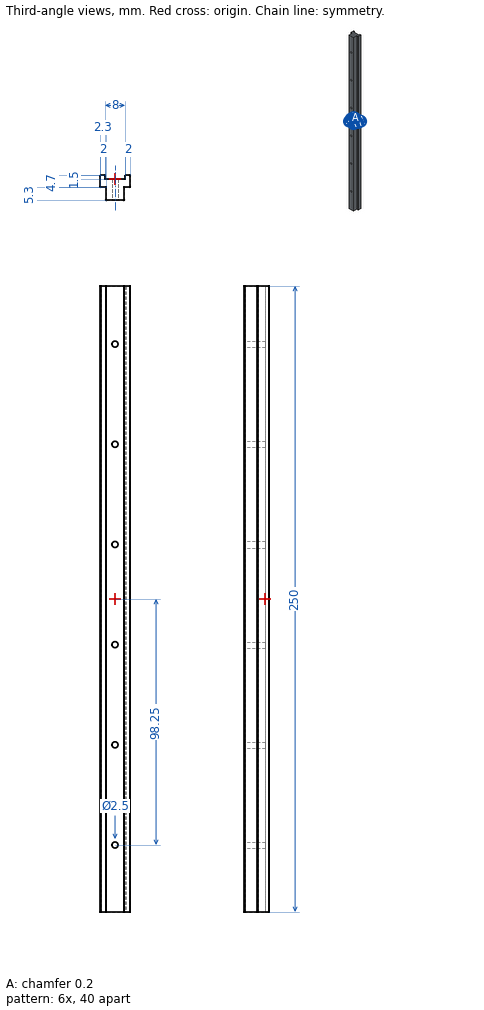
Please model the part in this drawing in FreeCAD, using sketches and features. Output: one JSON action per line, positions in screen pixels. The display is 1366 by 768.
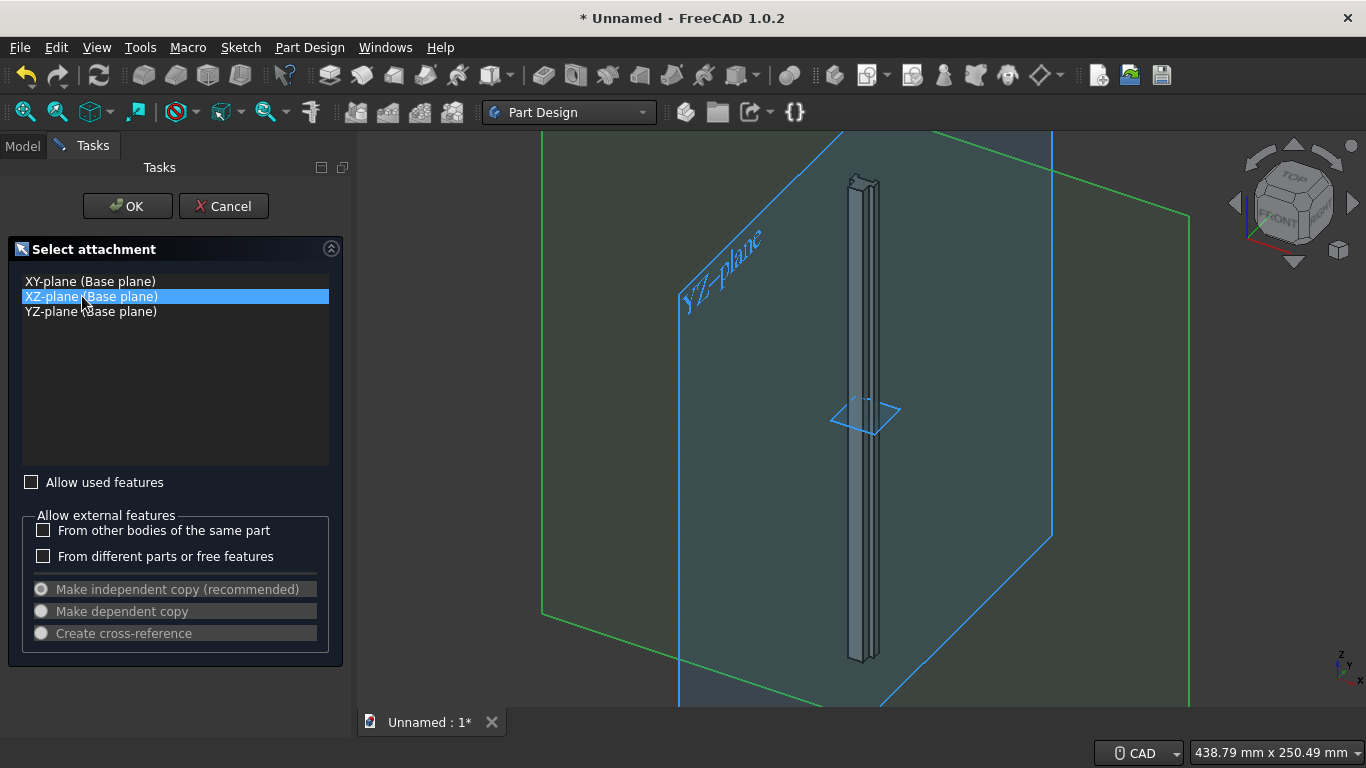
{"action": "left_click", "coordinate": [128, 206]}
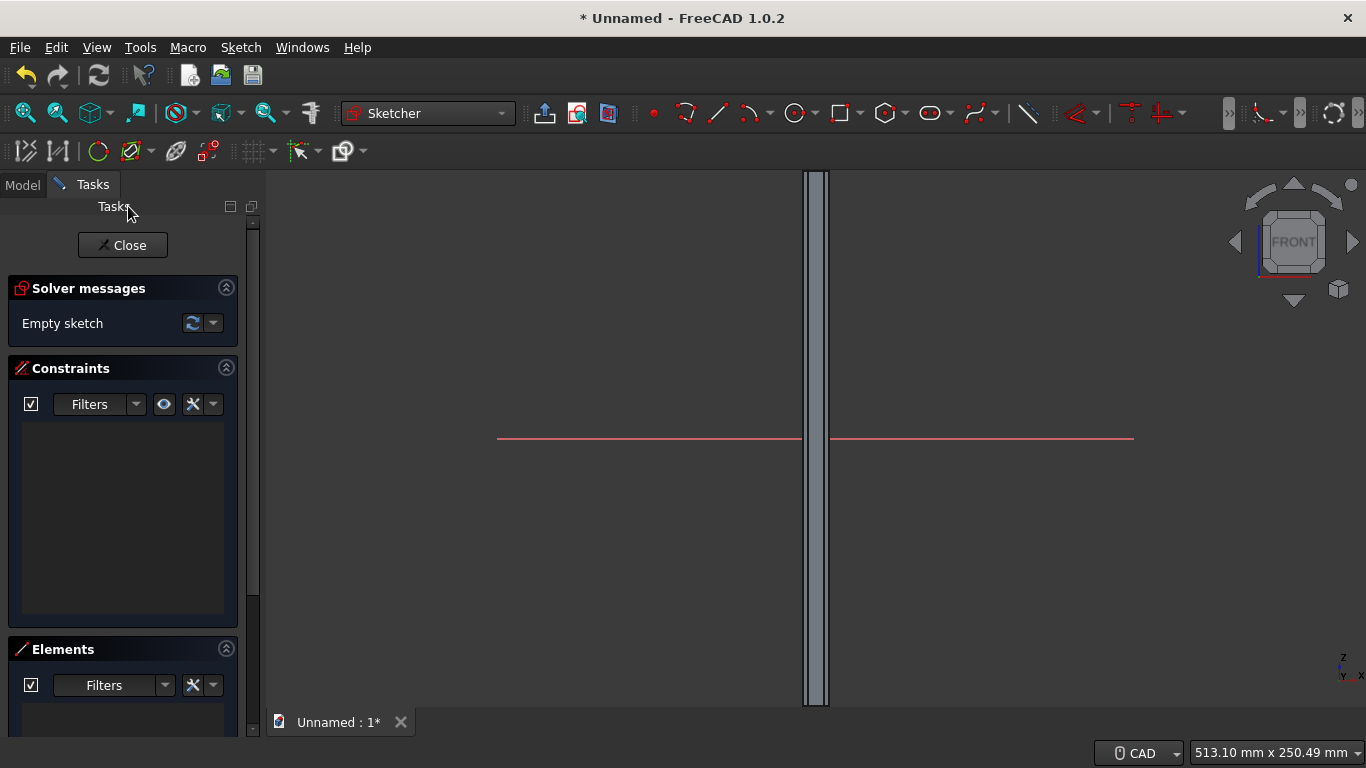
{"action": "key", "text": "q s"}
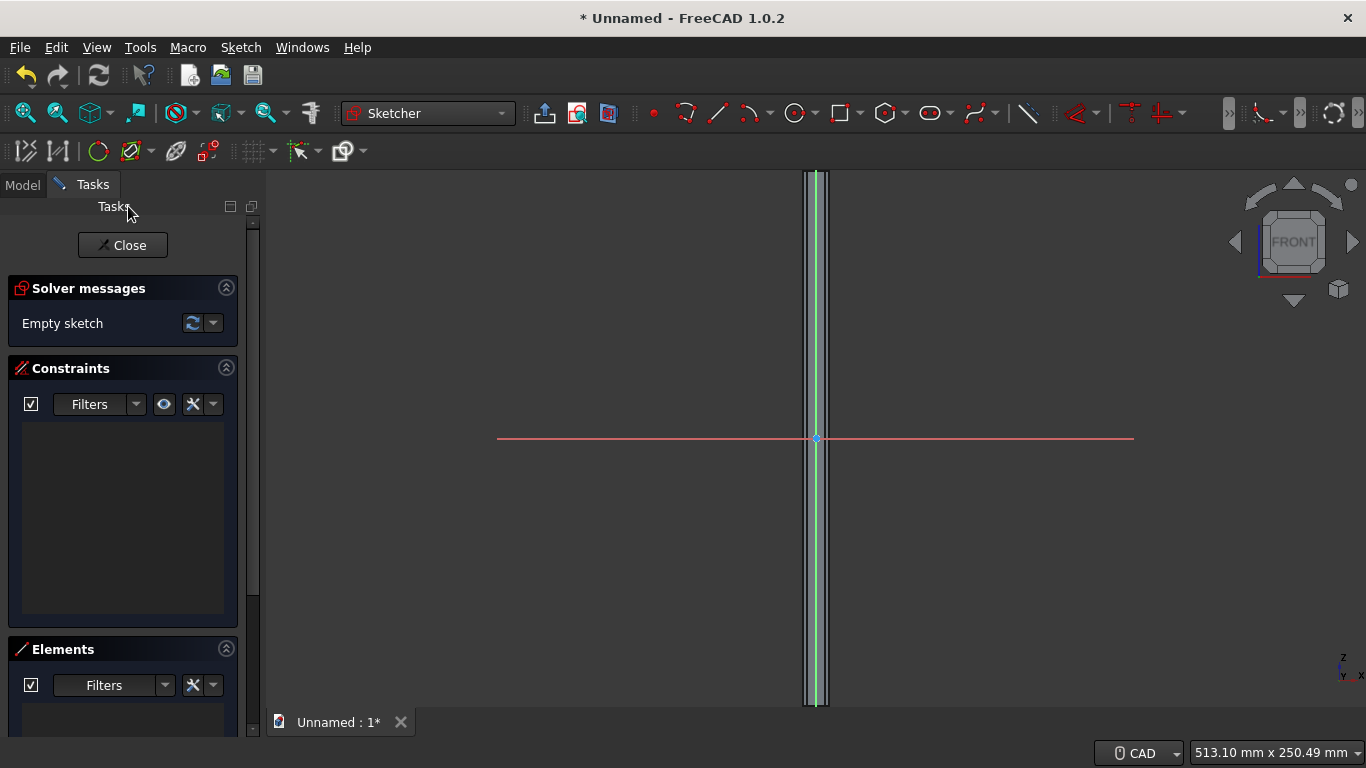
{"action": "scroll", "coordinate": [820, 660], "scroll_direction": "up", "scroll_amount": 15}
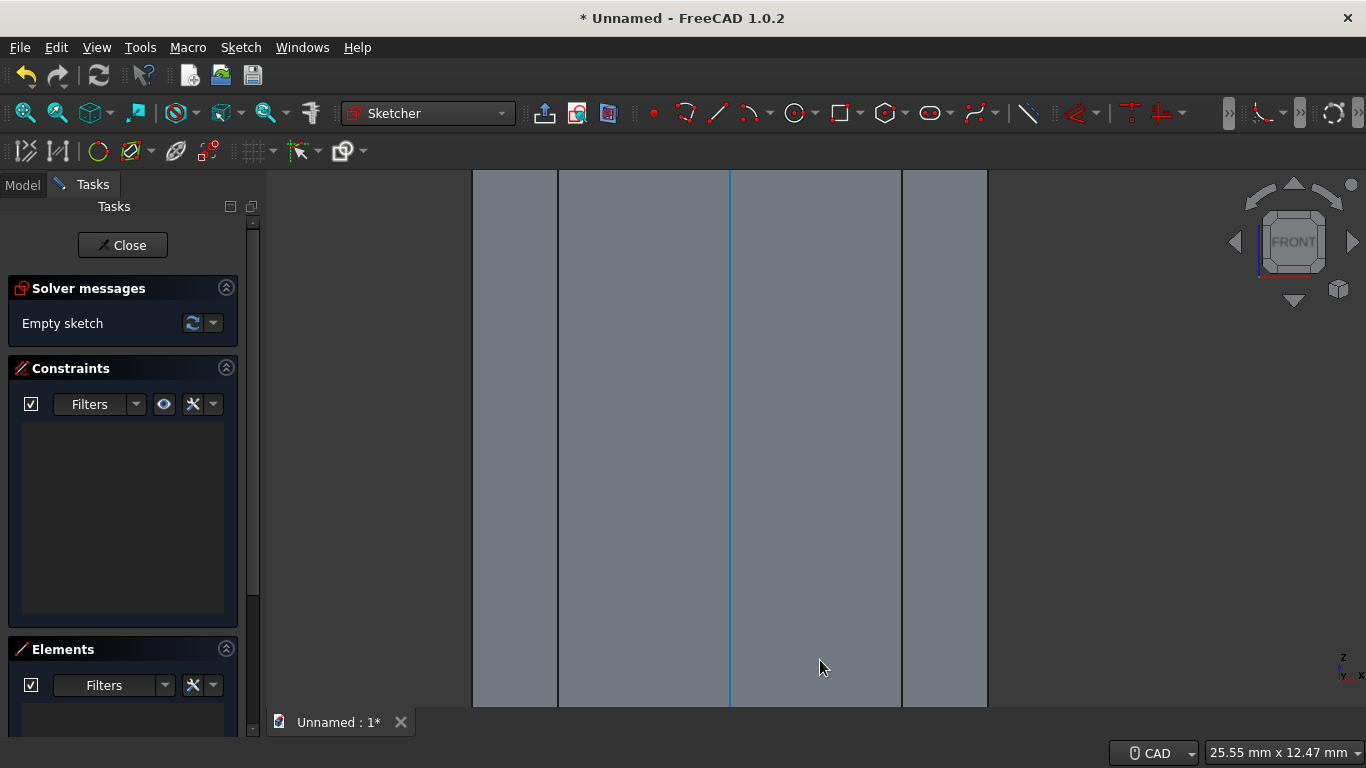
{"action": "scroll", "coordinate": [723, 418], "scroll_direction": "up", "scroll_amount": 6}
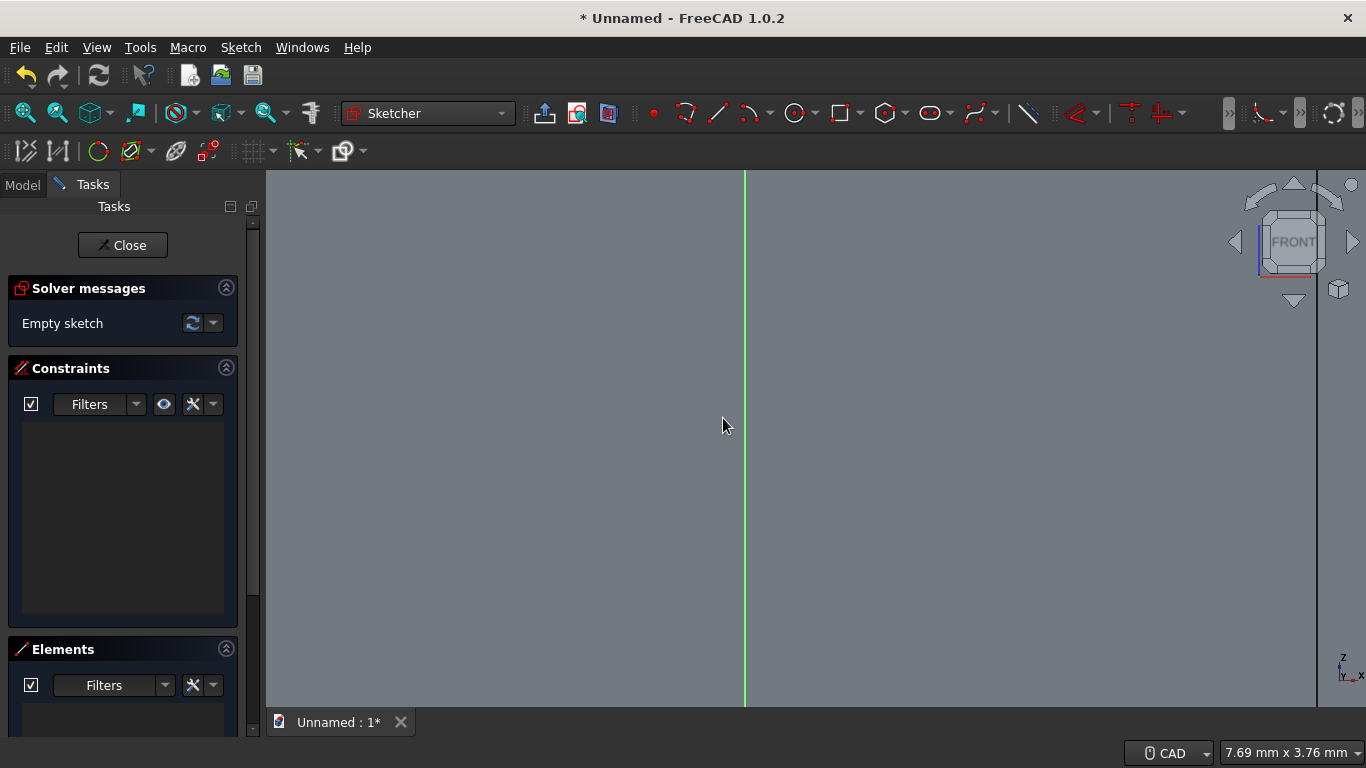
{"action": "left_click", "coordinate": [796, 114]}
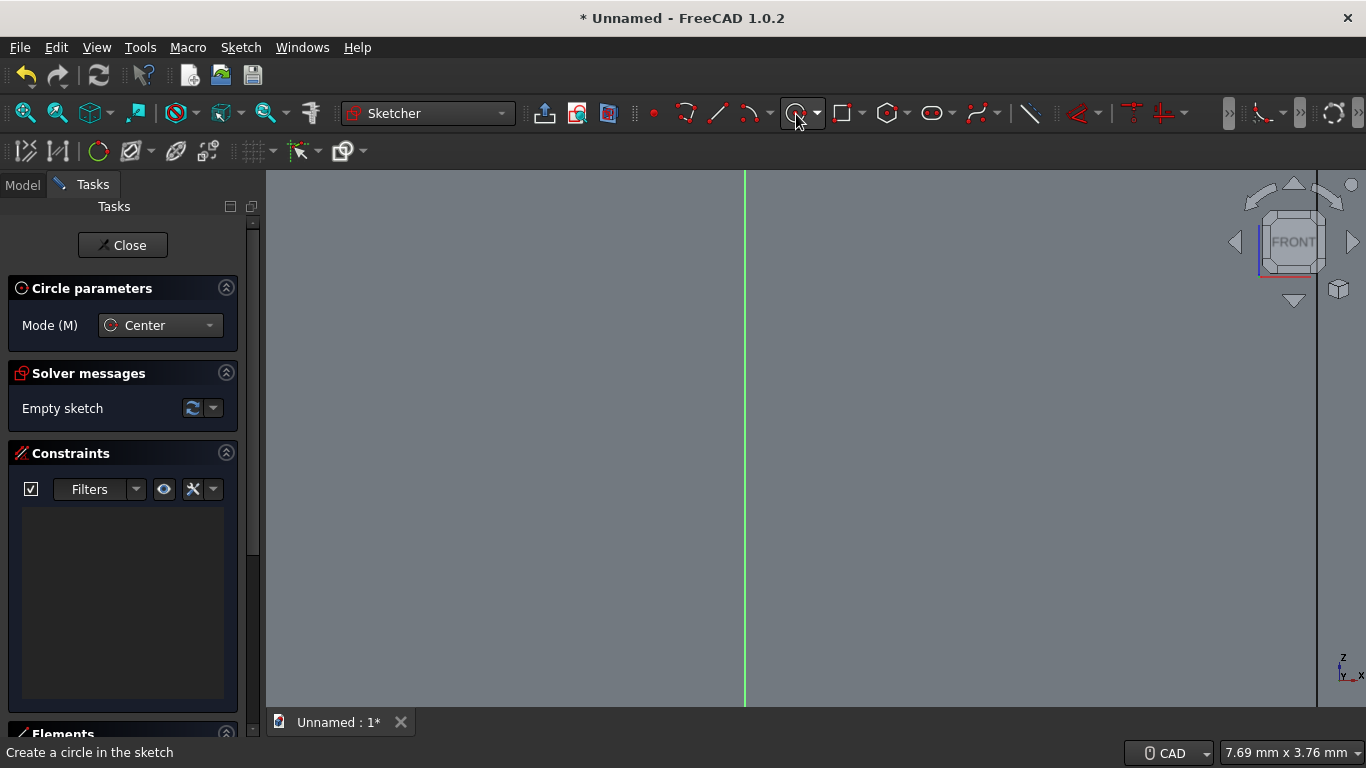
{"action": "left_click", "coordinate": [745, 438]}
{"action": "left_click", "coordinate": [872, 311]}
{"action": "key", "text": "Escape"}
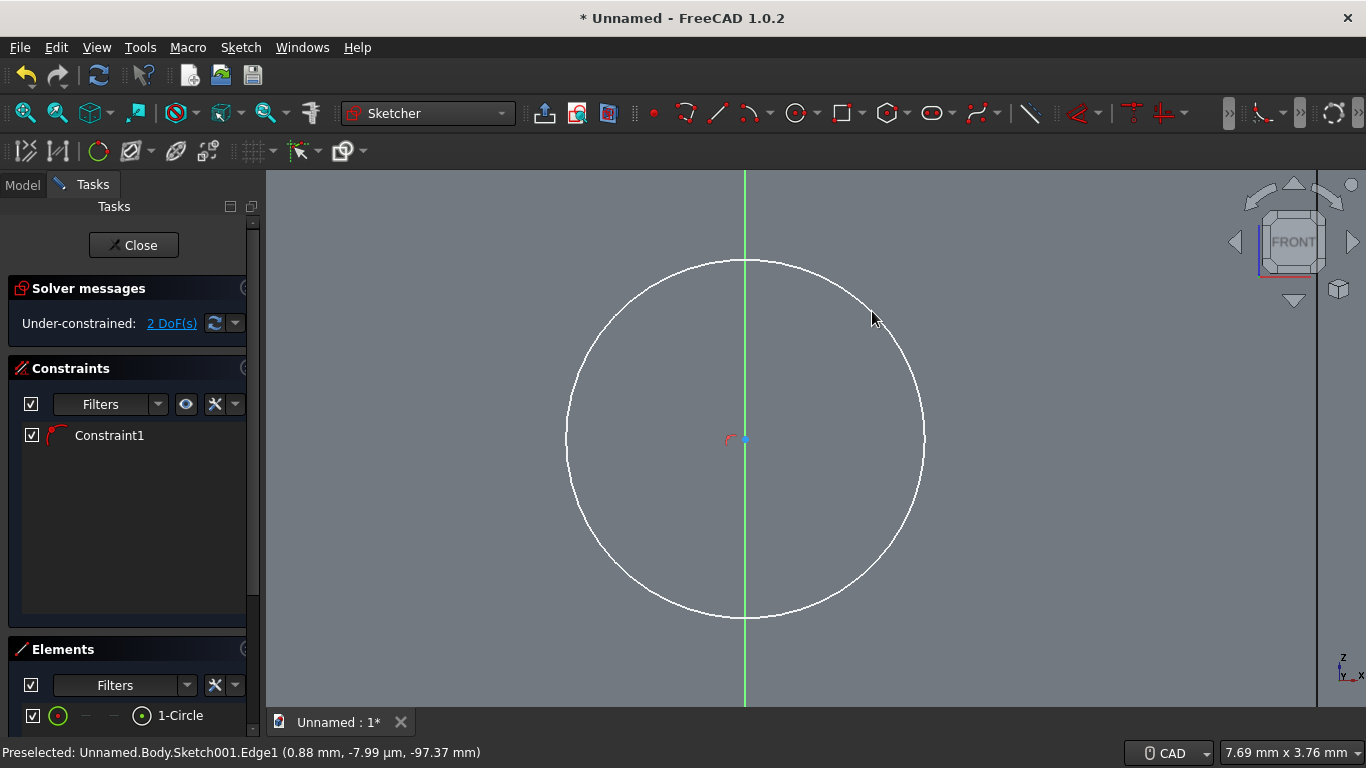
{"action": "left_click", "coordinate": [1078, 114]}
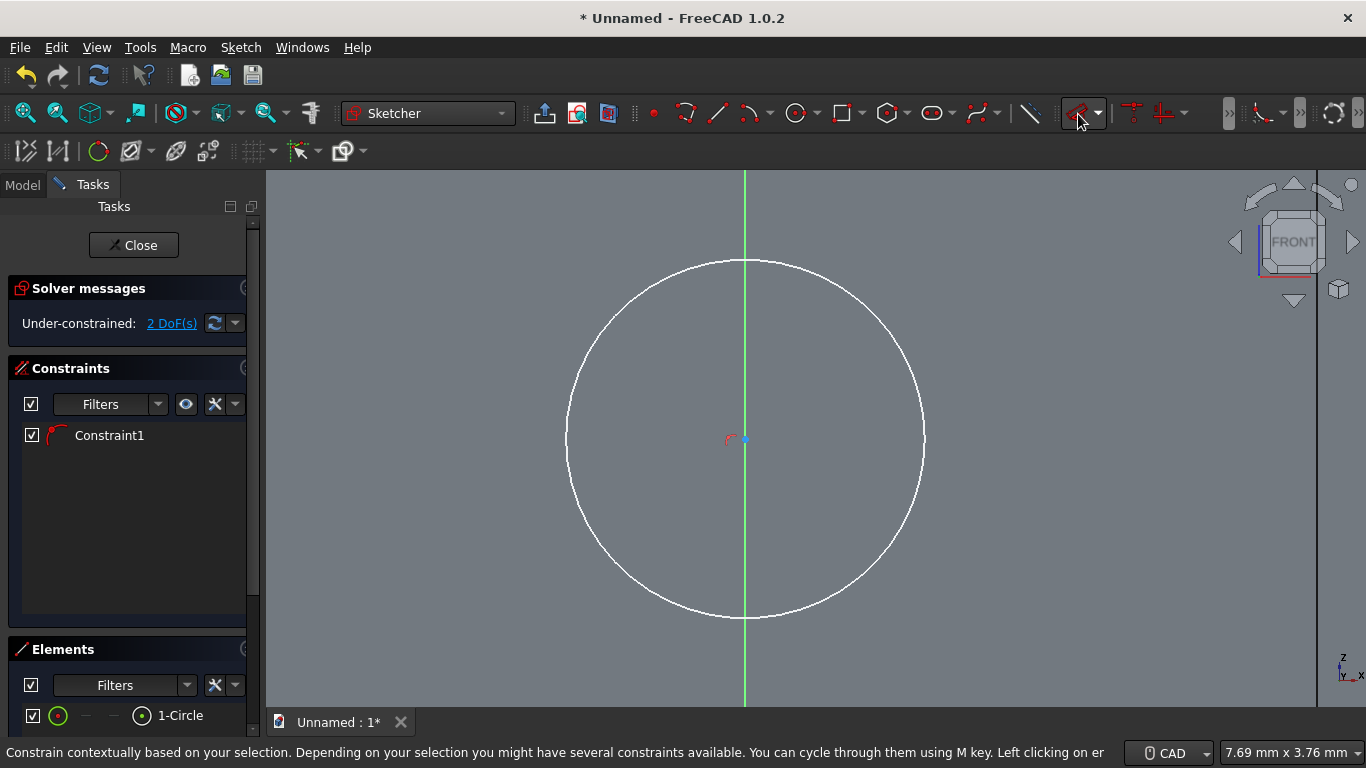
{"action": "left_click", "coordinate": [872, 312]}
{"action": "left_click", "coordinate": [895, 289]}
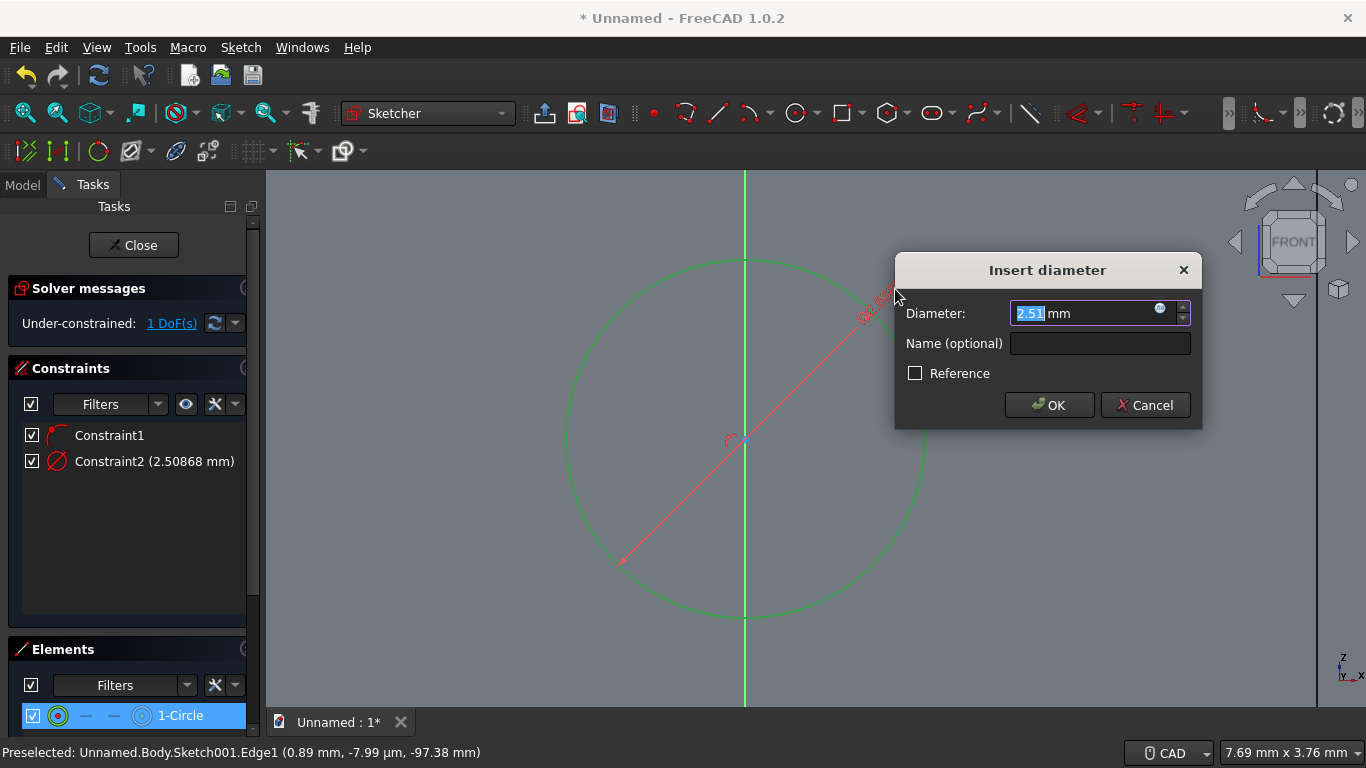
{"action": "type", "text": "2.5"}
{"action": "key", "text": "Return"}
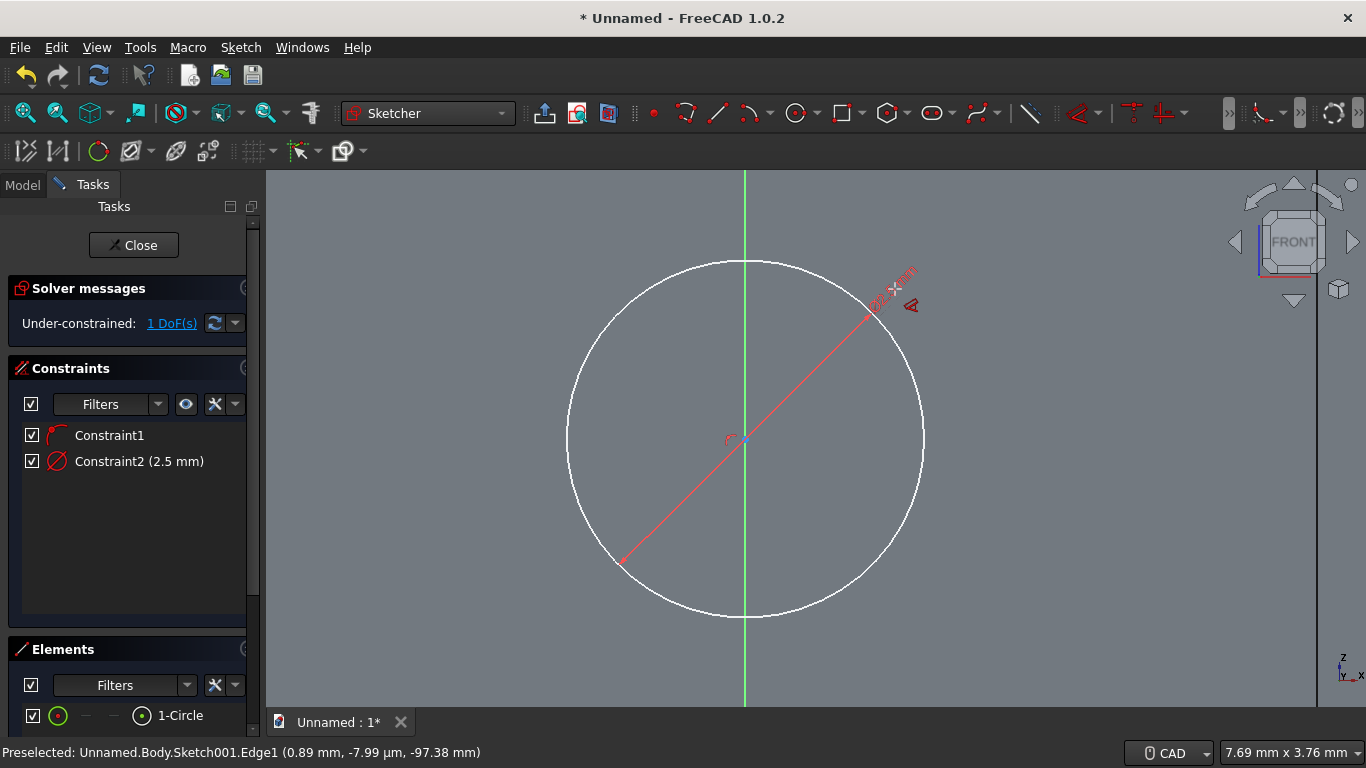
{"action": "left_click", "coordinate": [745, 439]}
{"action": "left_click", "coordinate": [779, 318]}